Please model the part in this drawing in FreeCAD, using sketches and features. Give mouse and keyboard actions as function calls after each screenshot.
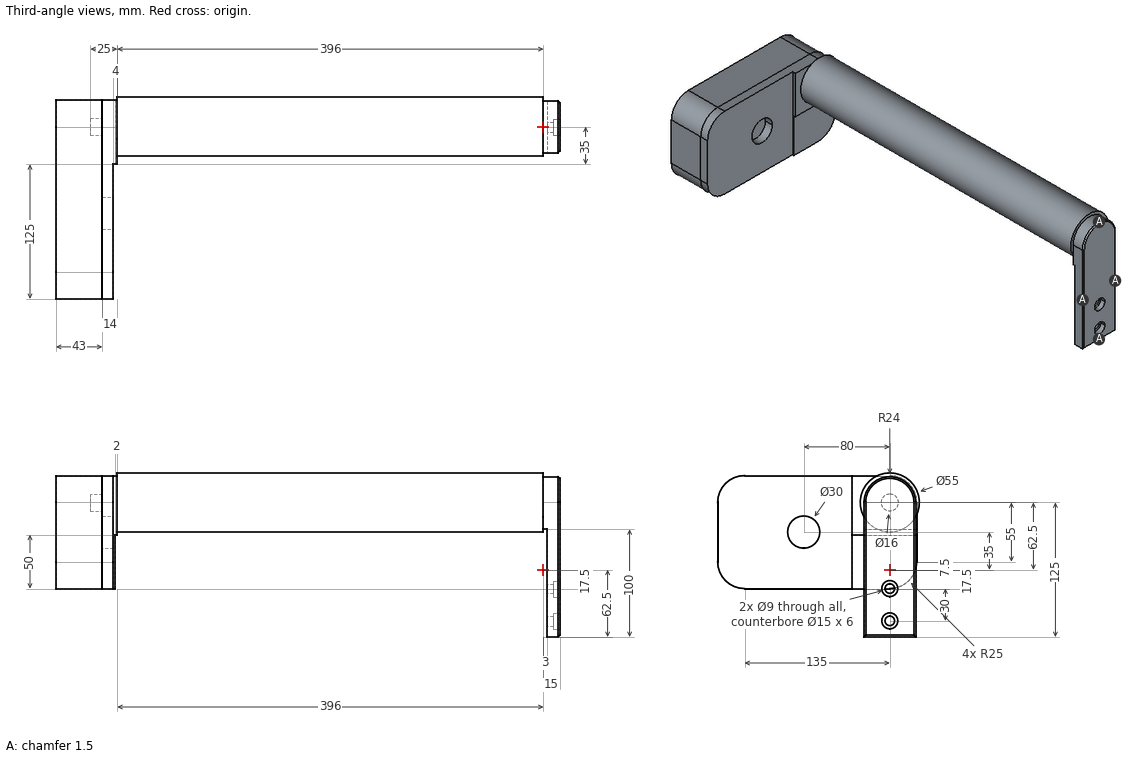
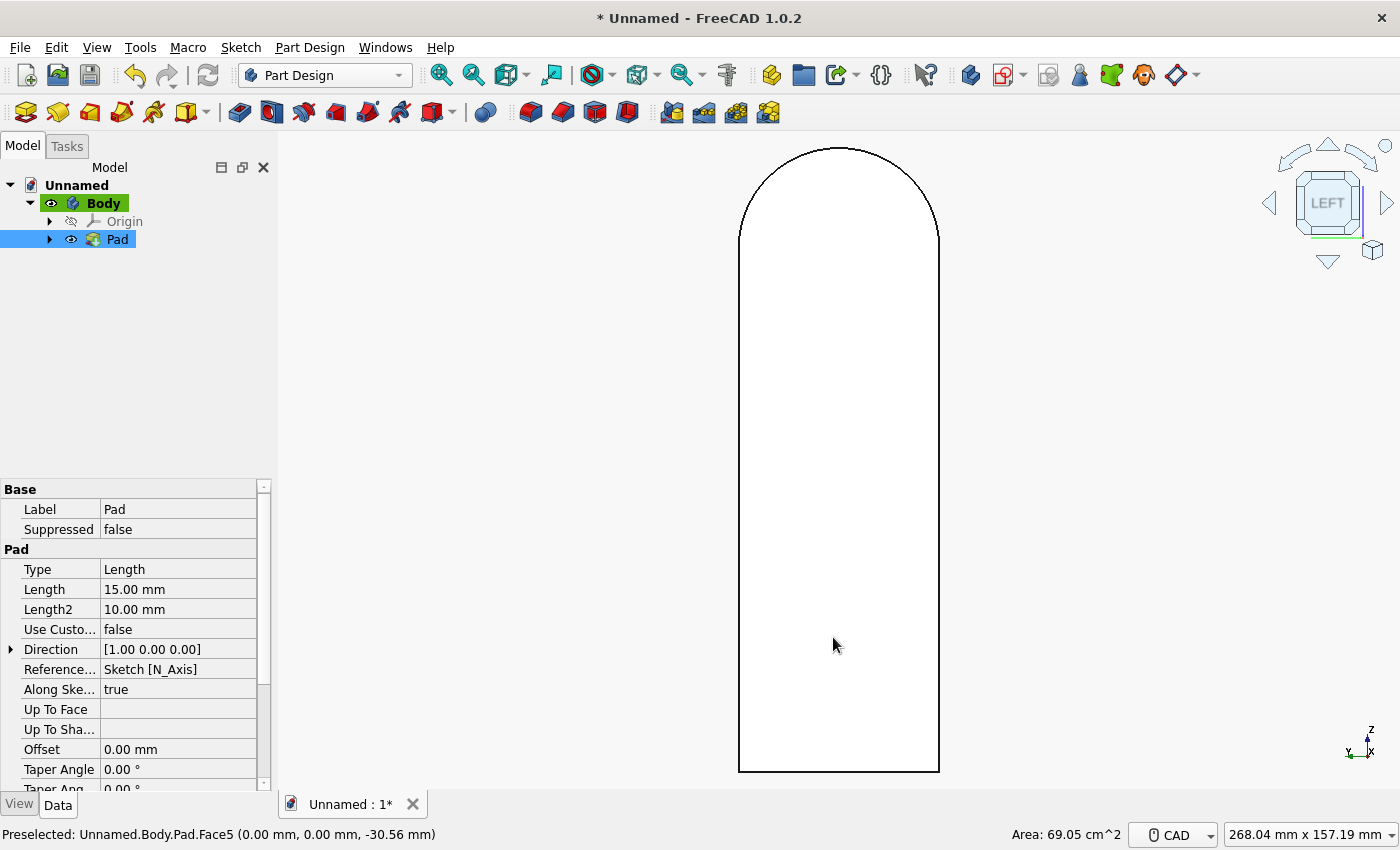
click(1004, 76)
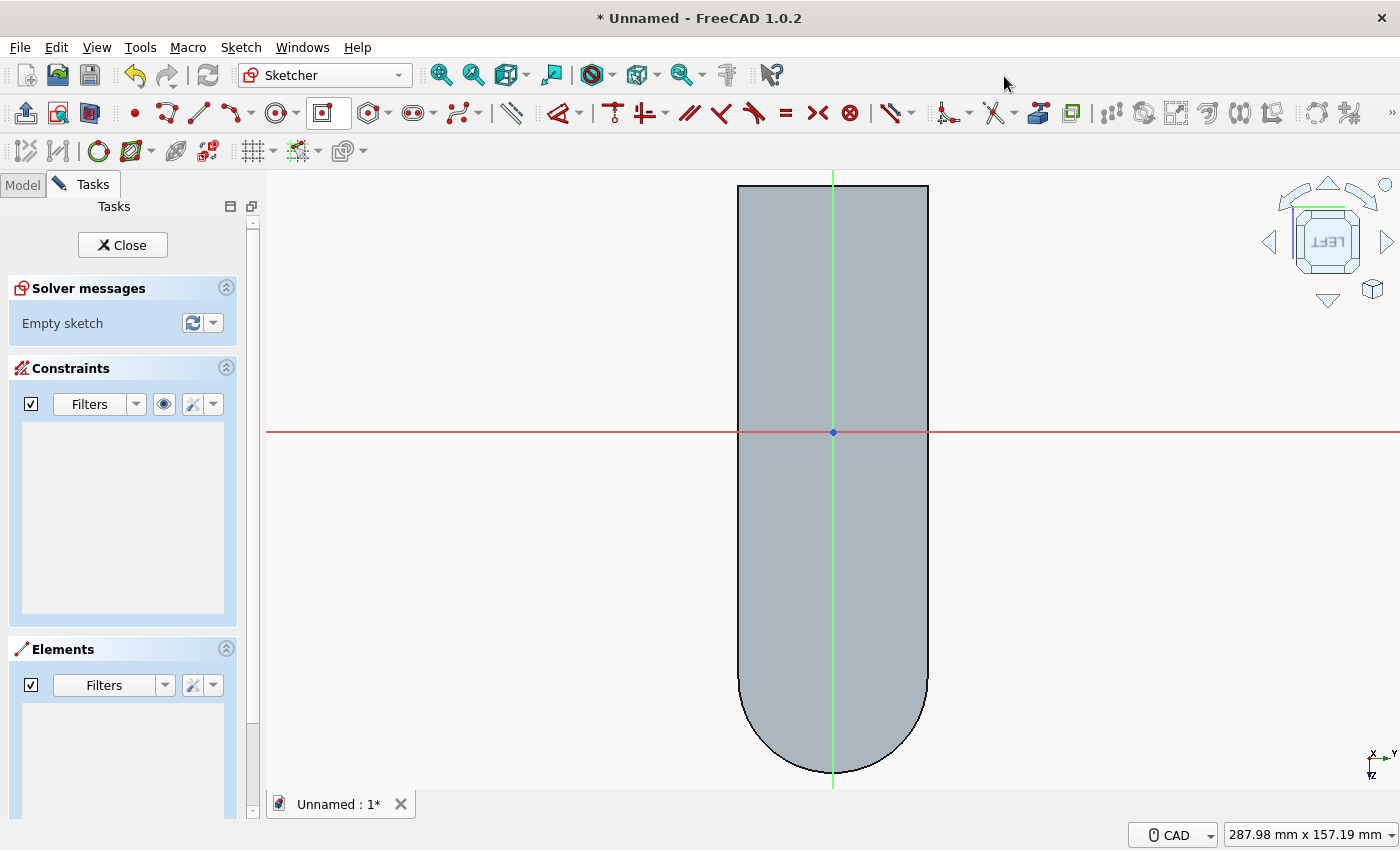
scroll(455, 198, down, 1)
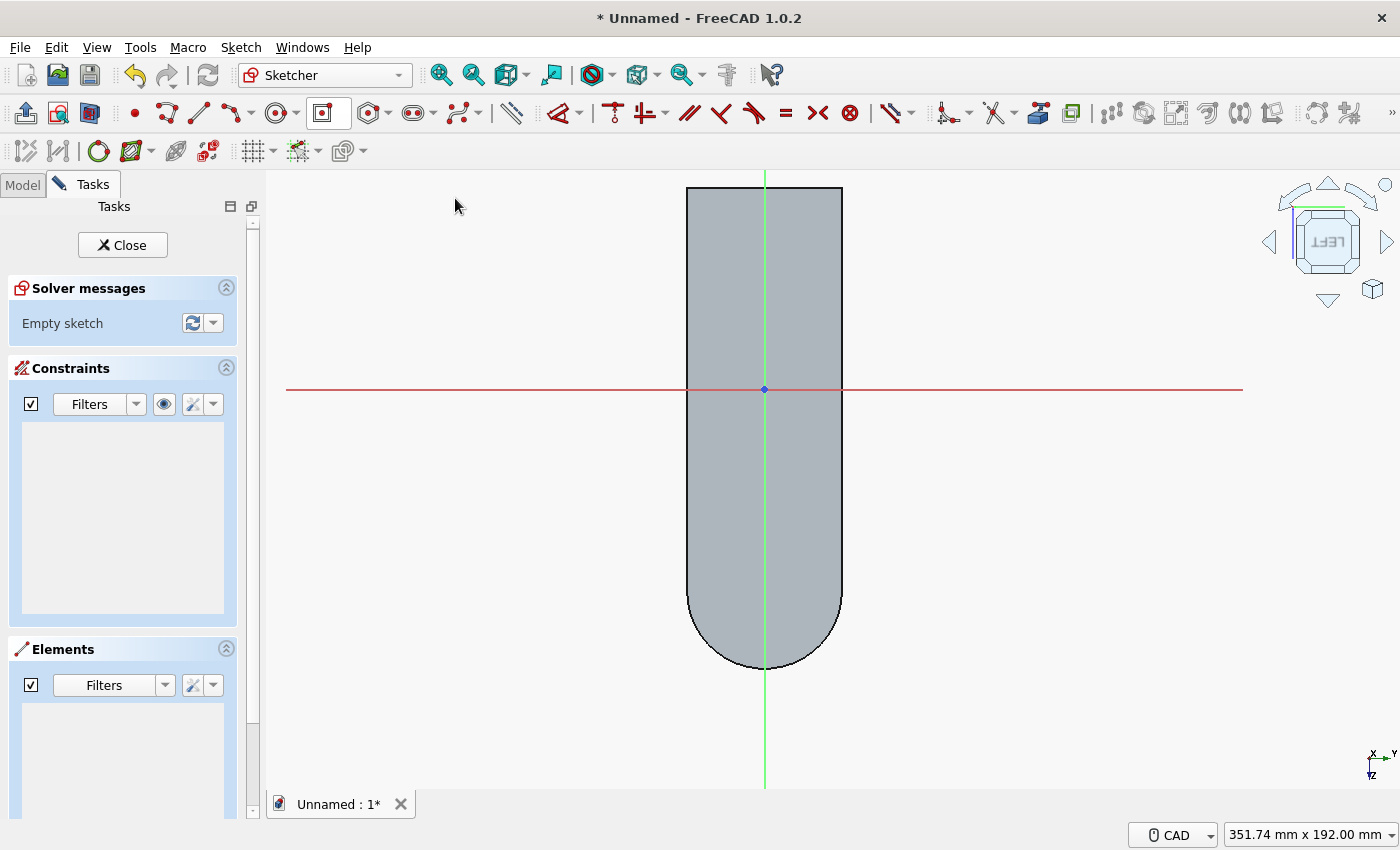
scroll(765, 648, up, 2)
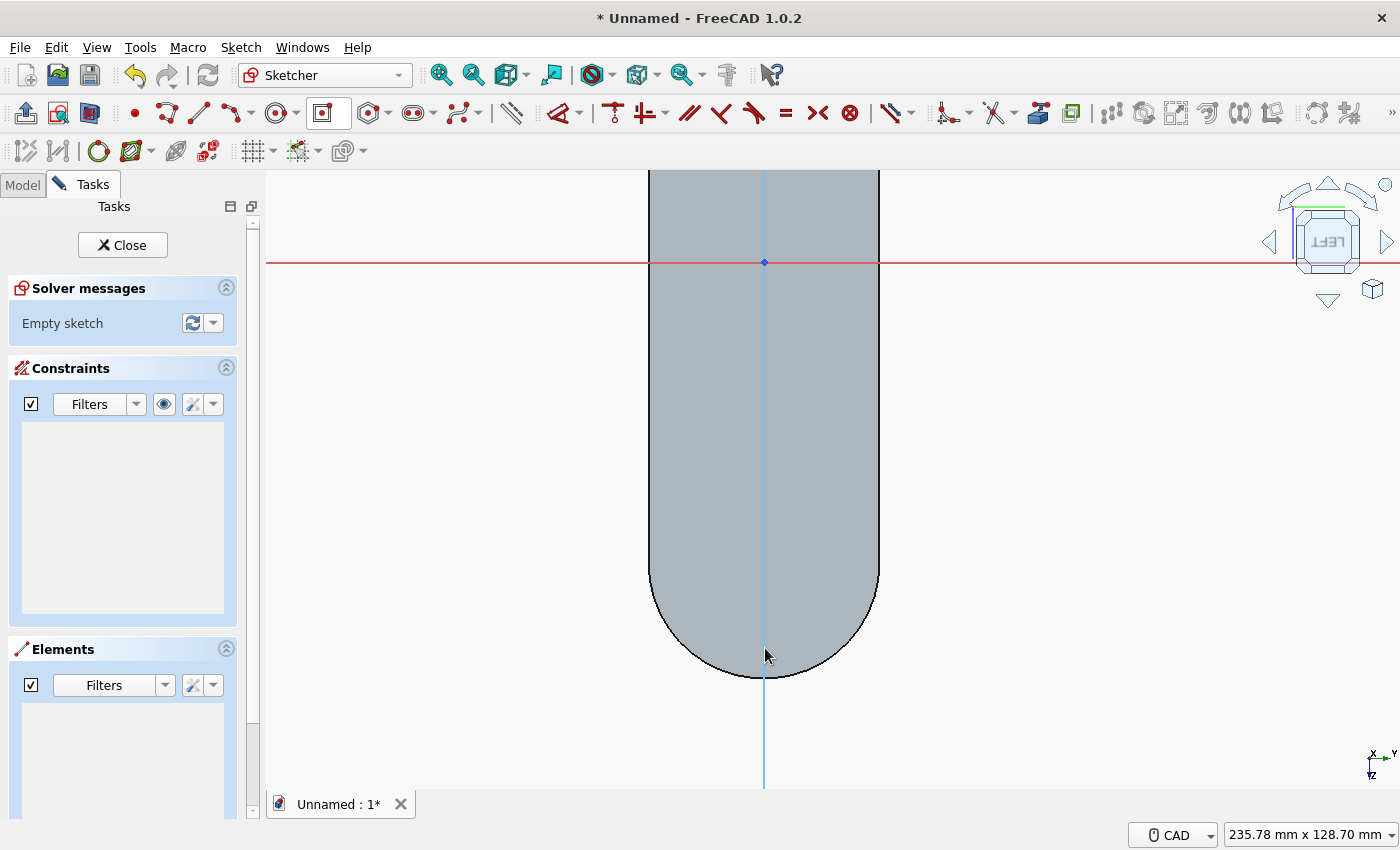
key(g)
key(c)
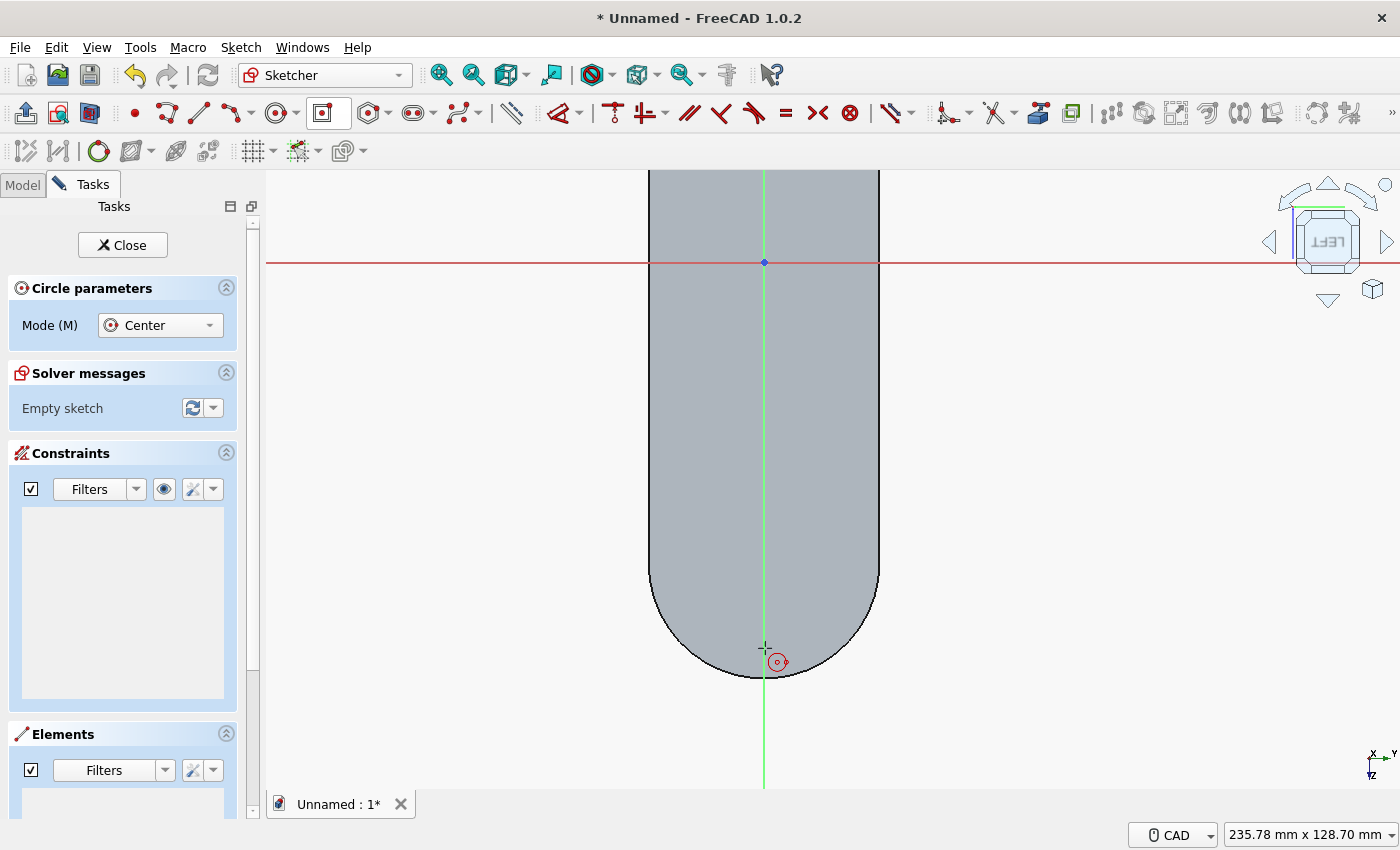
click(764, 563)
move(858, 470)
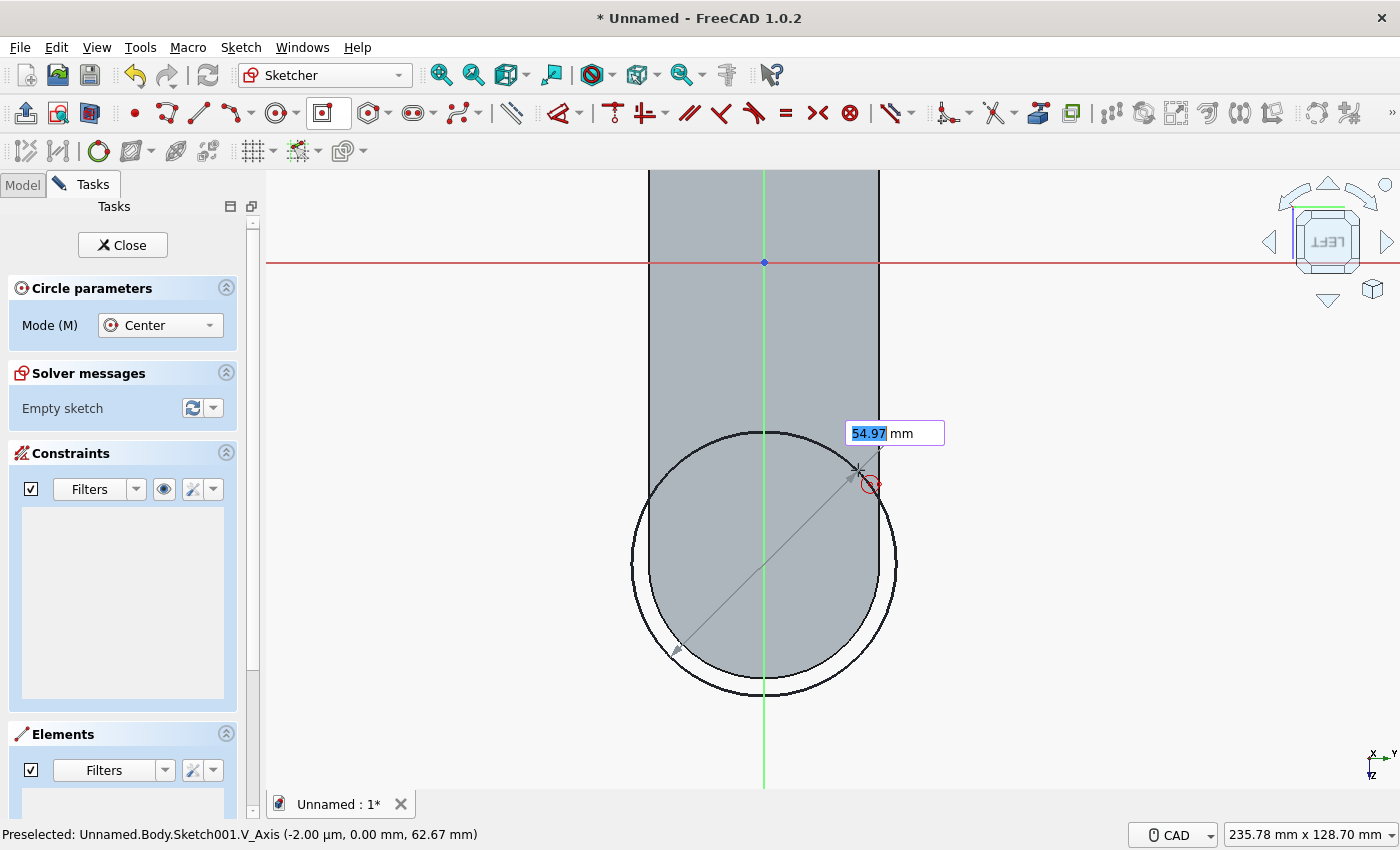
text(55)
key(Return)
key(Escape)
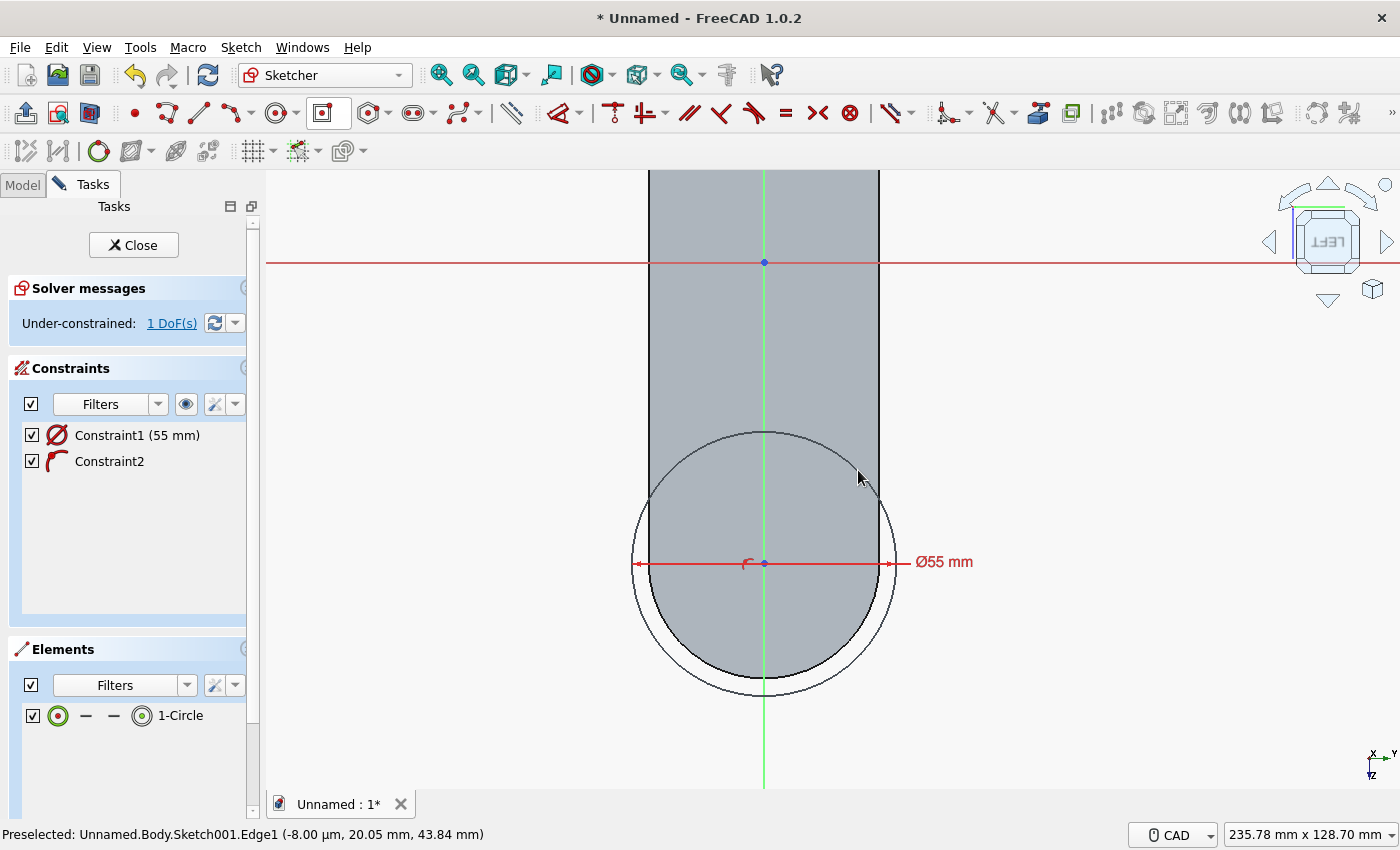
click(558, 114)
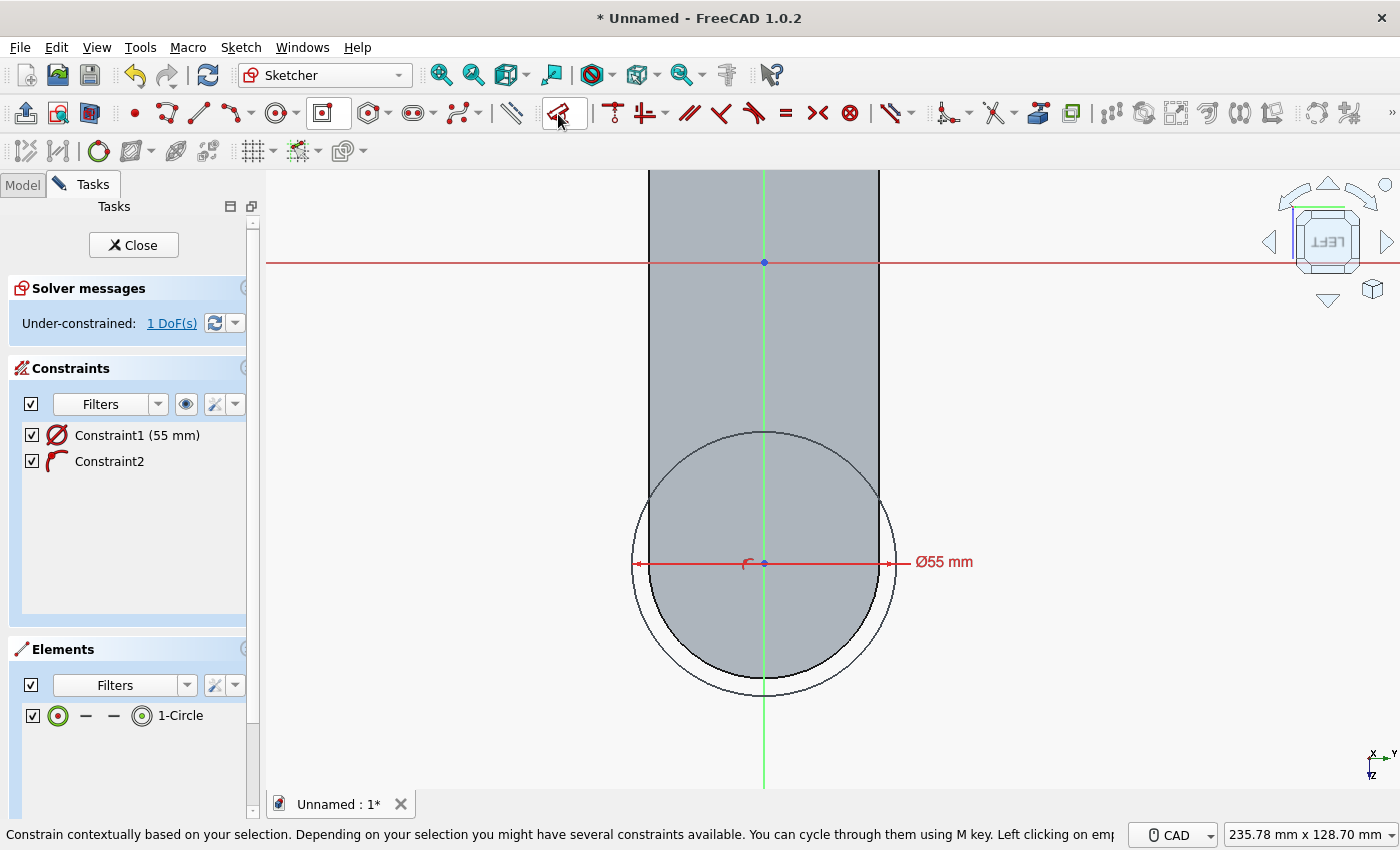
click(764, 564)
click(798, 413)